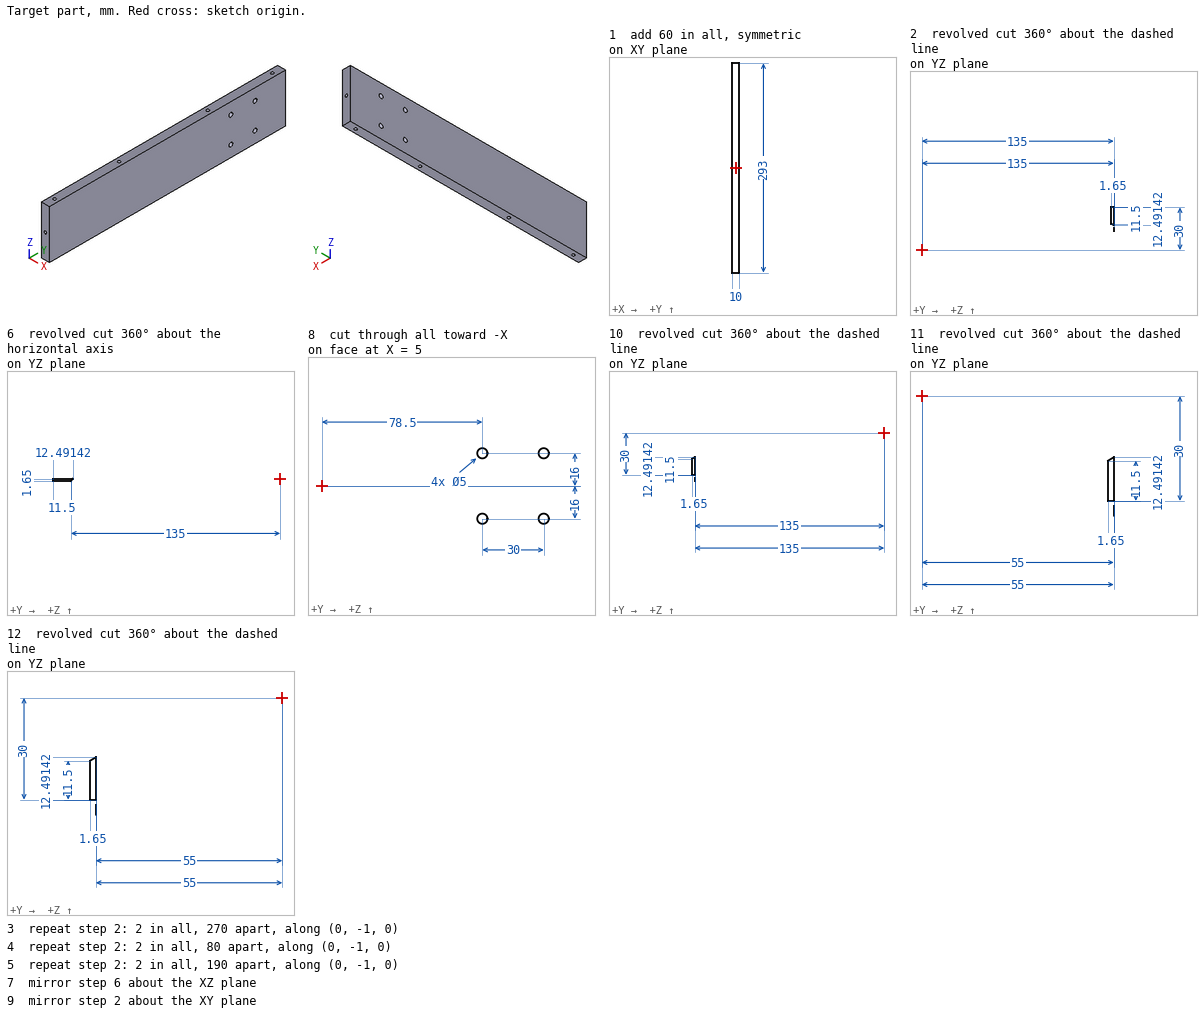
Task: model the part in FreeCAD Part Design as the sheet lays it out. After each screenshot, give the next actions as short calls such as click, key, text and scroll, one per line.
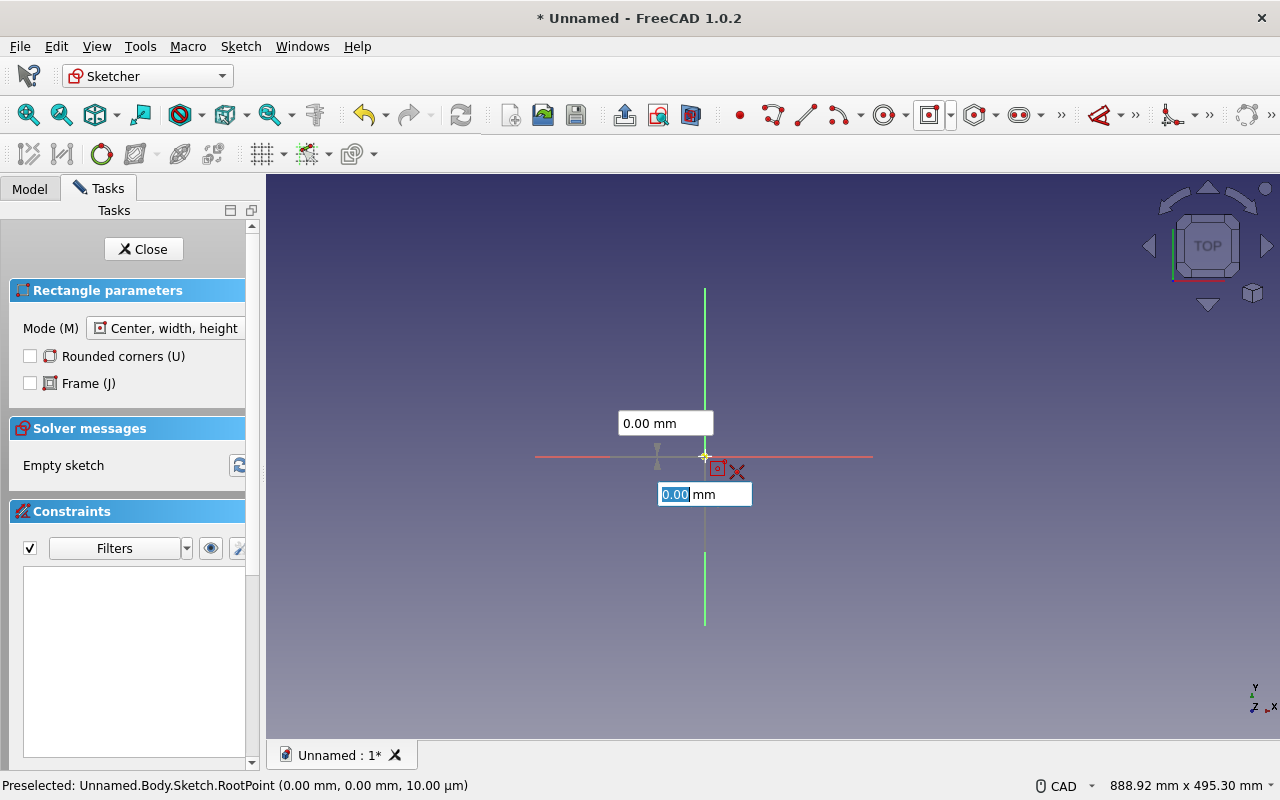
scroll(710, 289, up, 6)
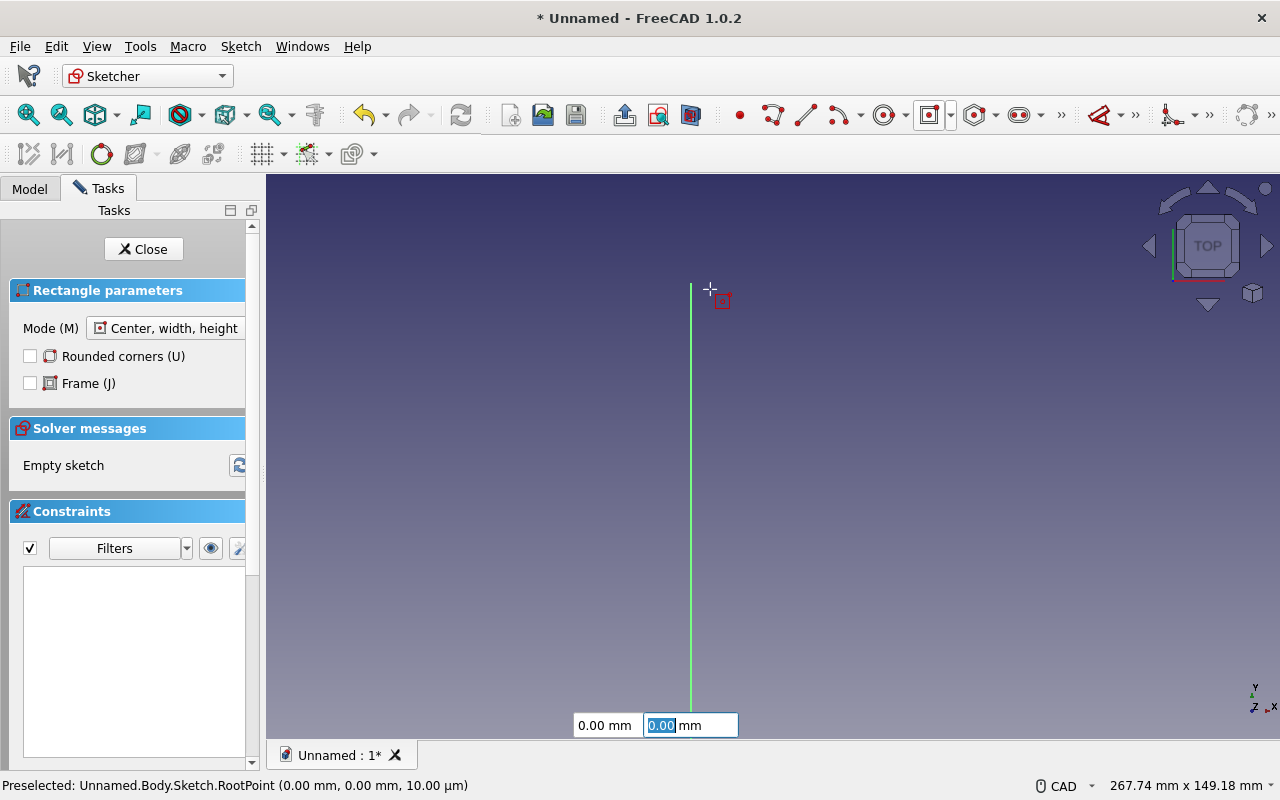
click(710, 290)
key(Escape)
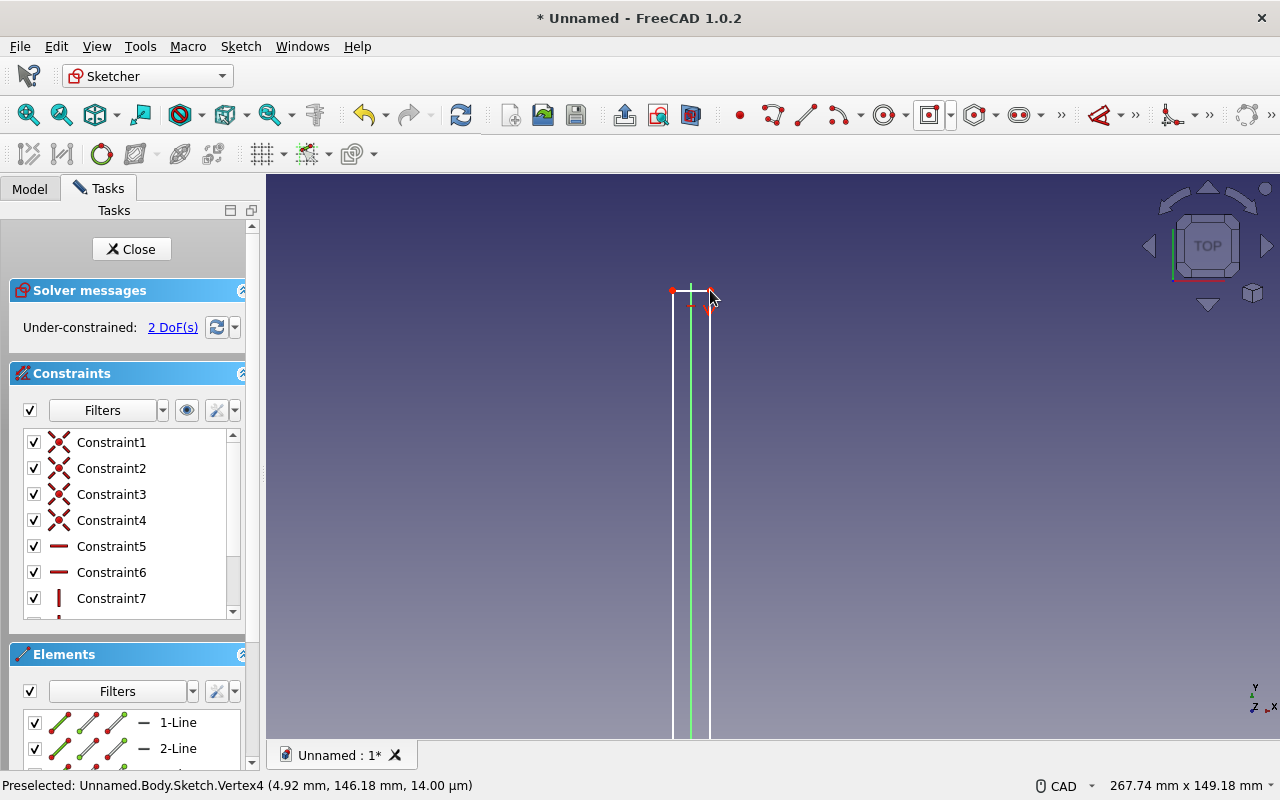
scroll(710, 289, down, 6)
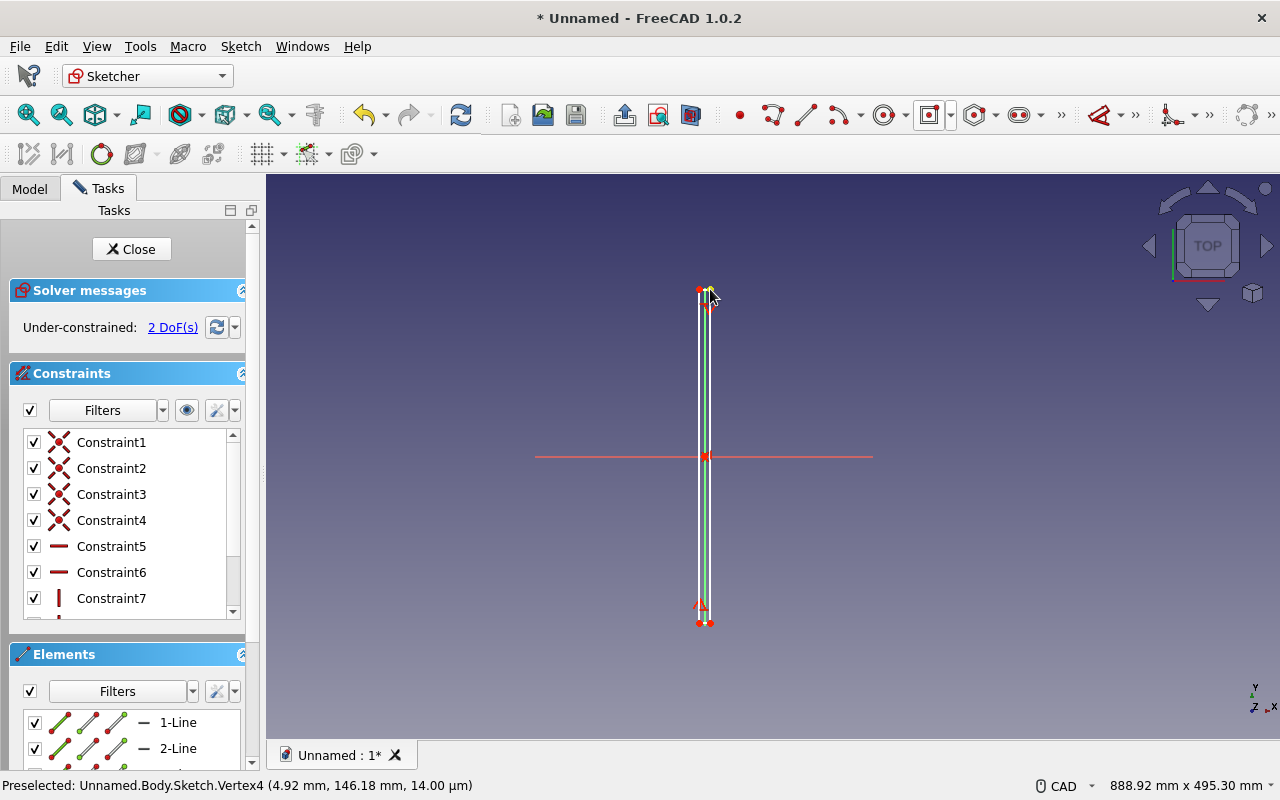
scroll(704, 623, up, 7)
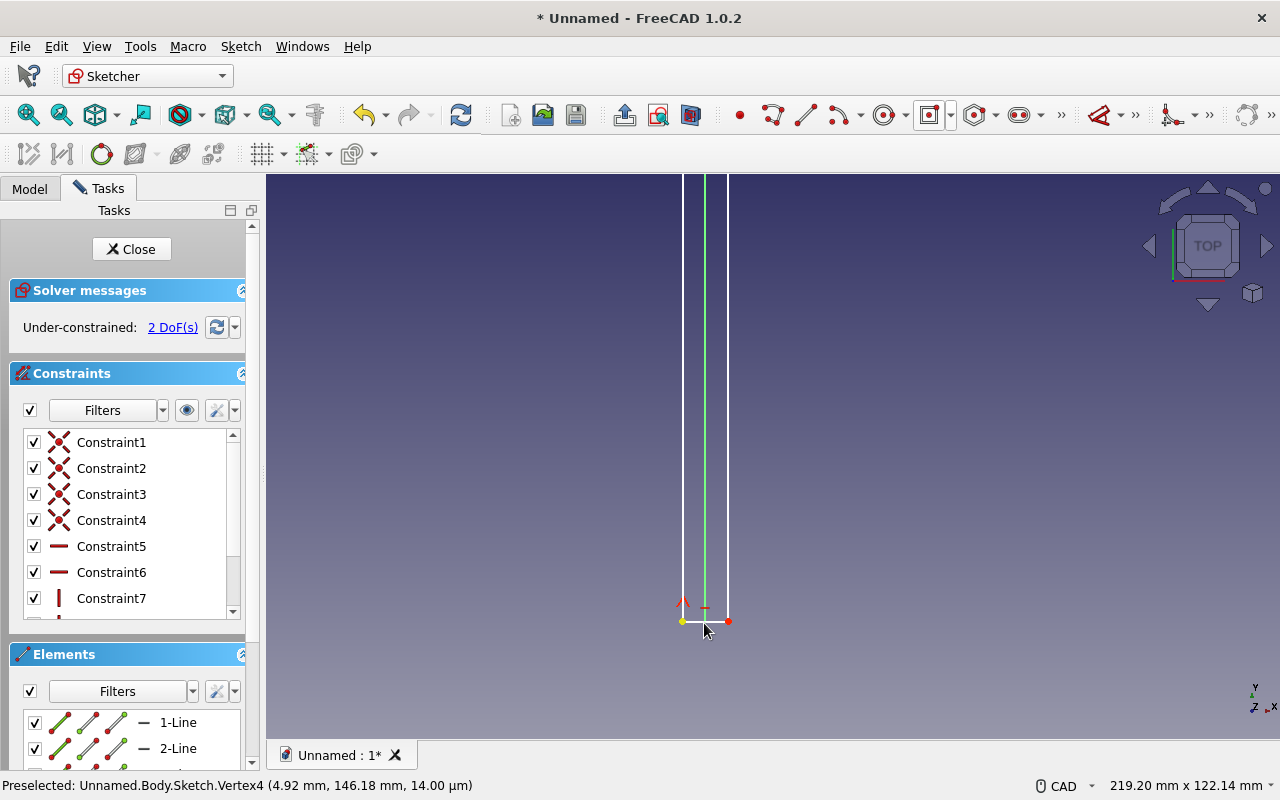
click(701, 622)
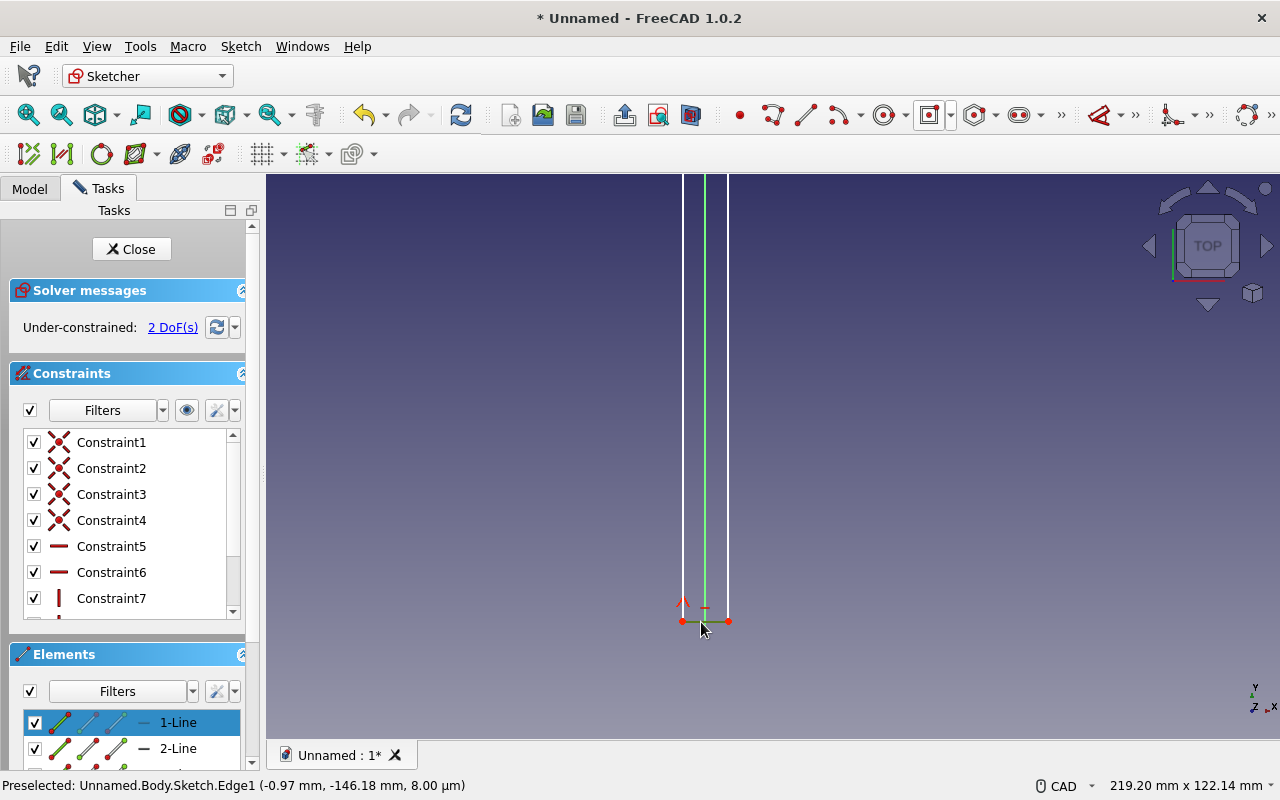
key(l)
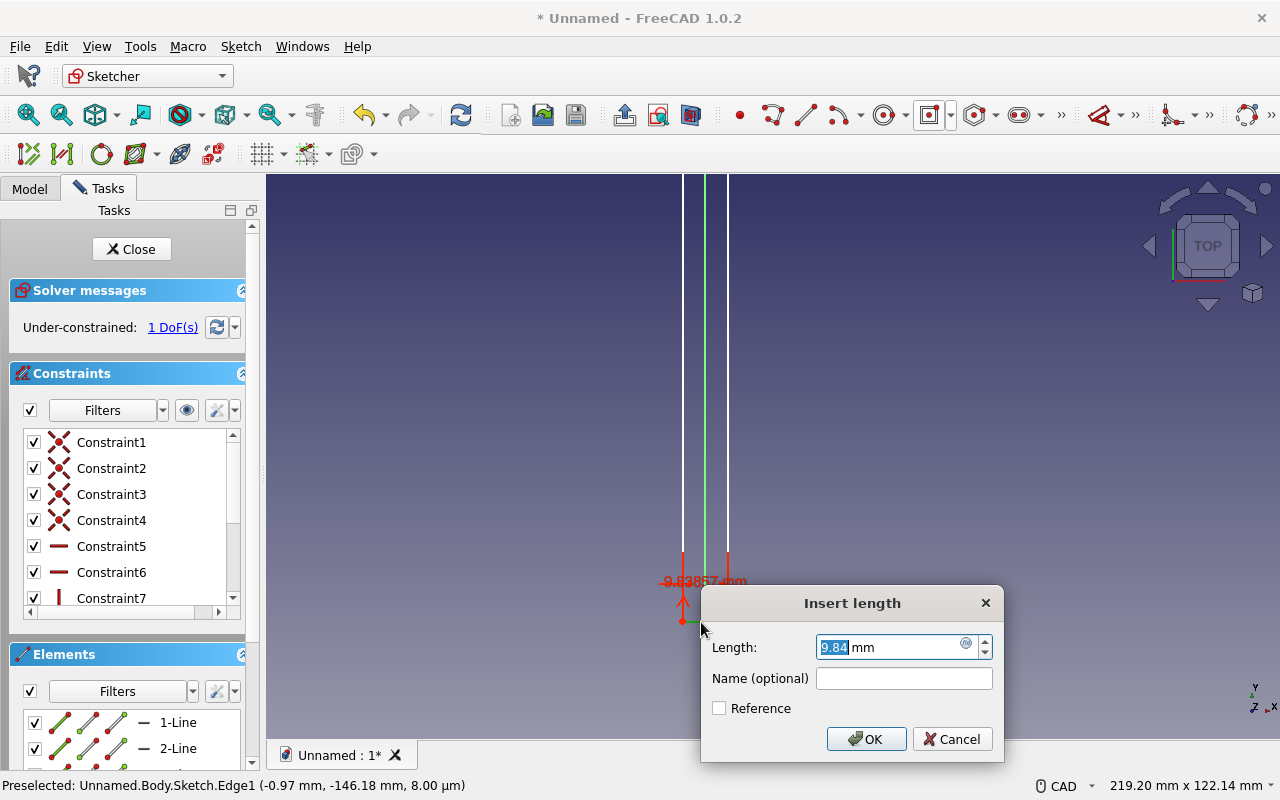
text(10)
key(Return)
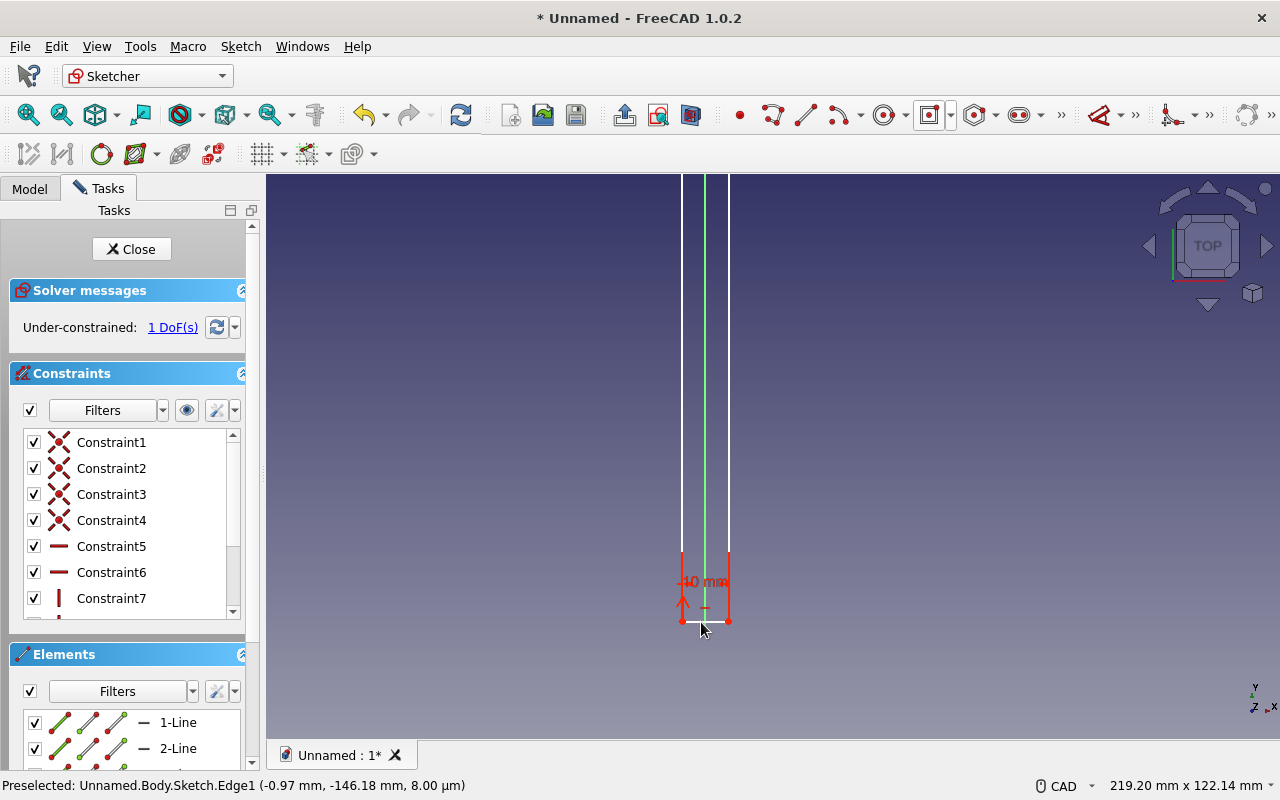
click(729, 216)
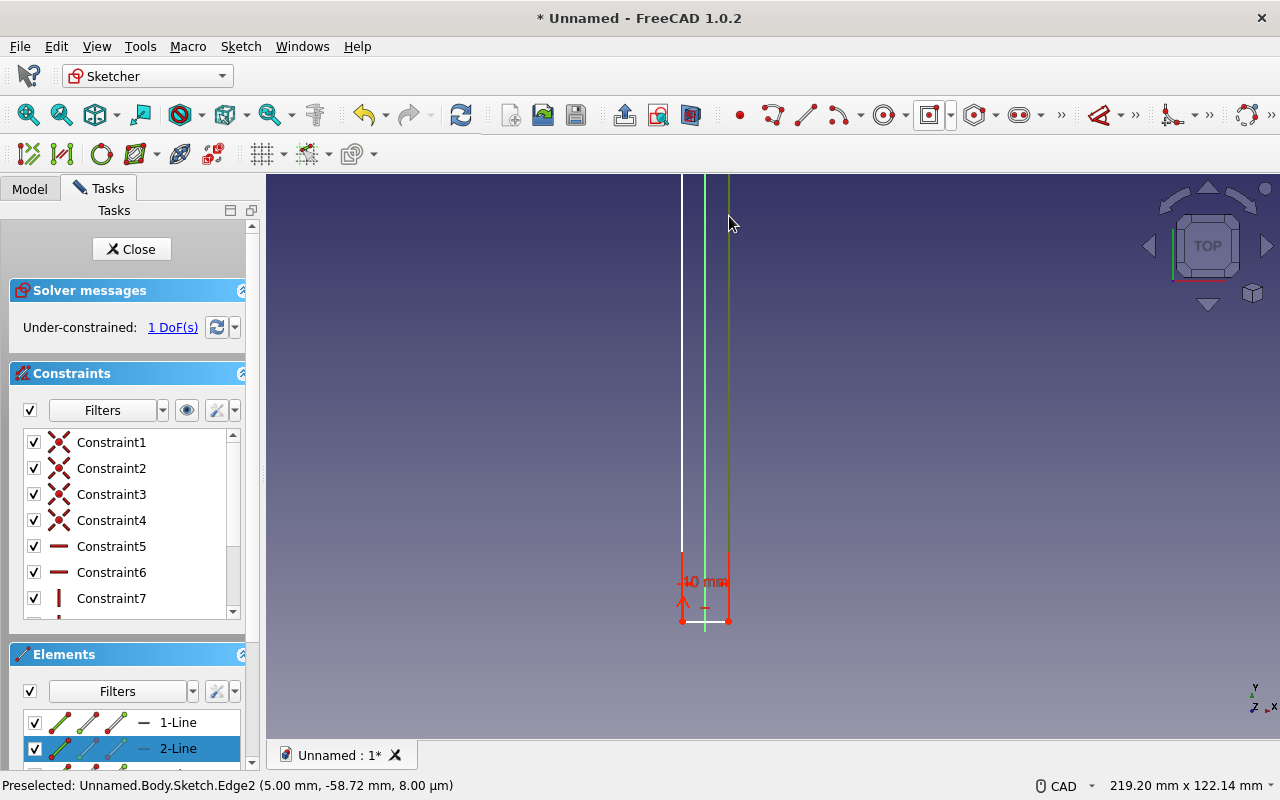
key(i)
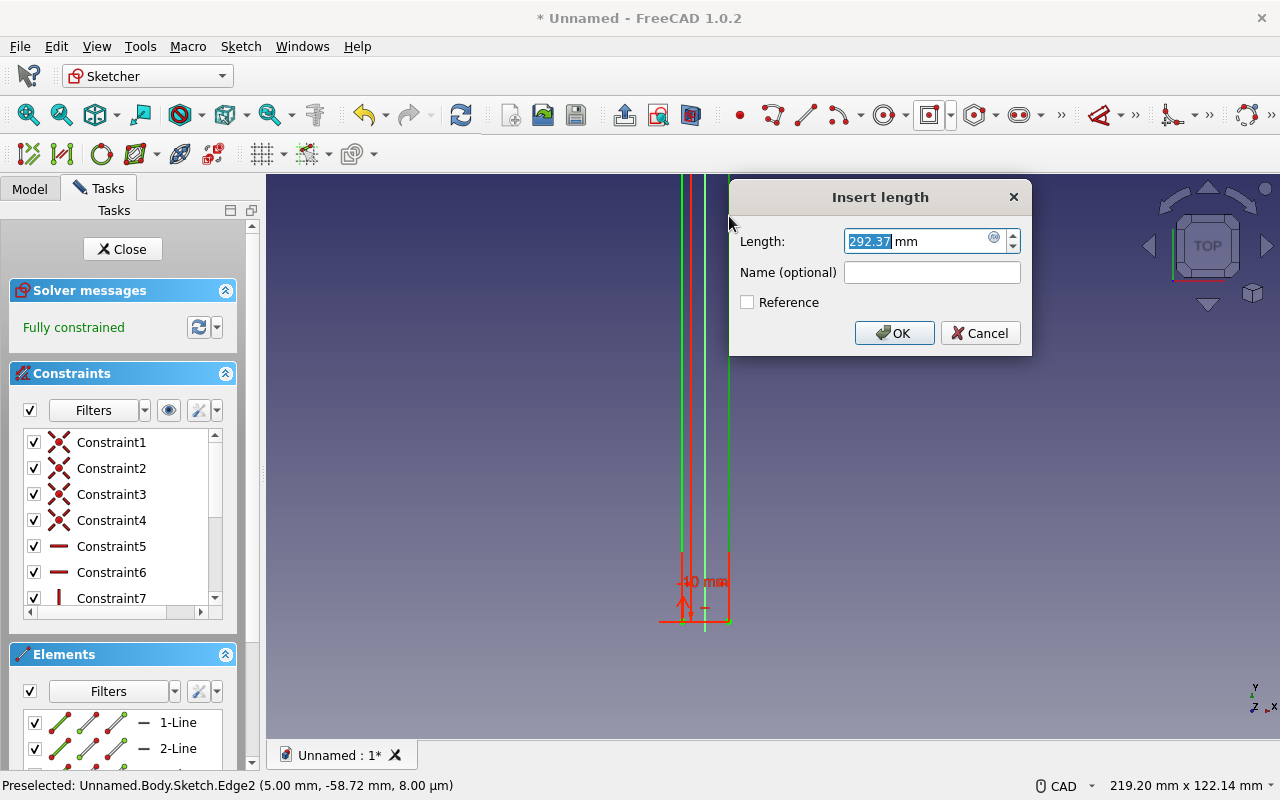
text(293)
key(Return)